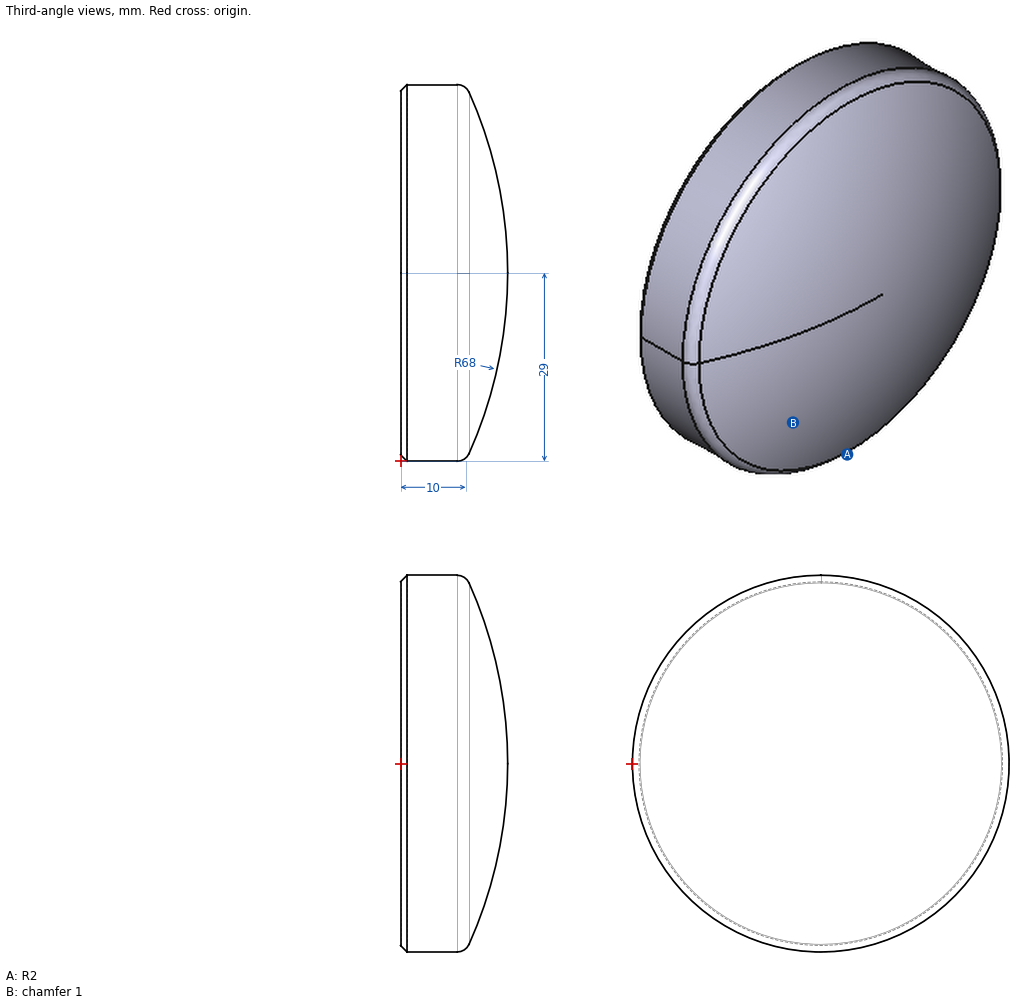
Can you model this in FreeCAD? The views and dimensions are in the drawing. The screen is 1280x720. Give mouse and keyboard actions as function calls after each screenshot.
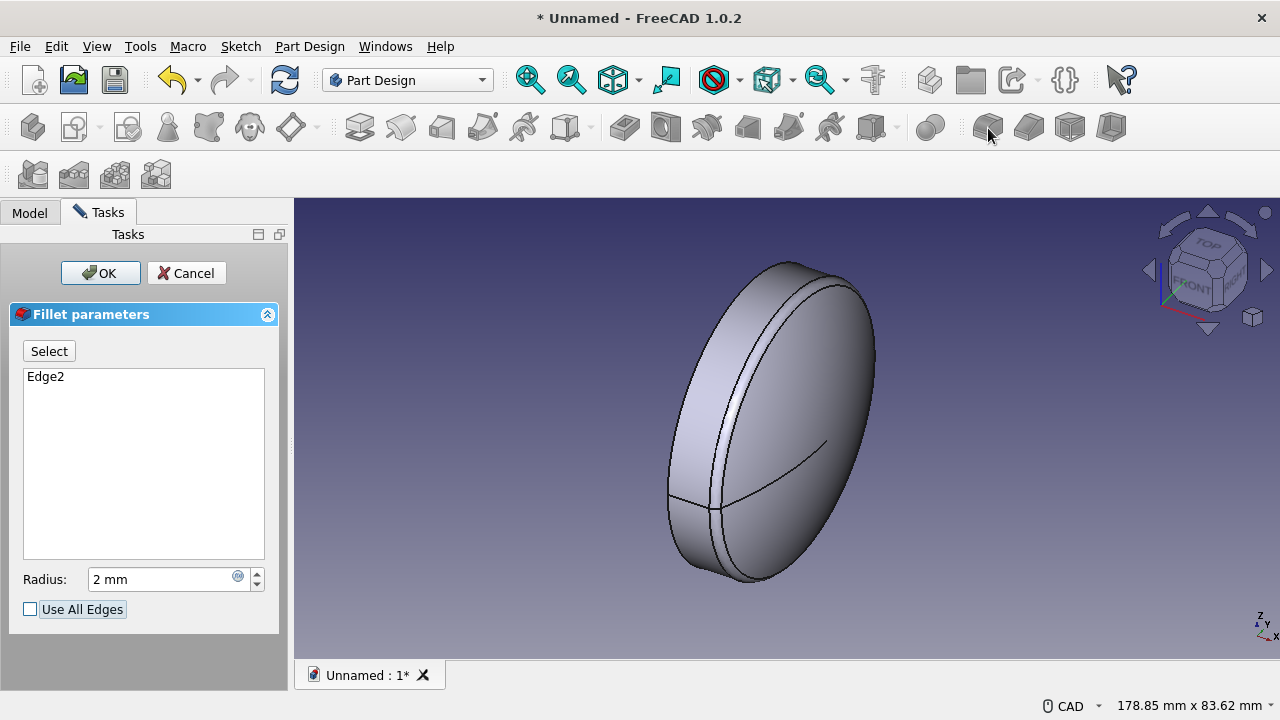
click(101, 273)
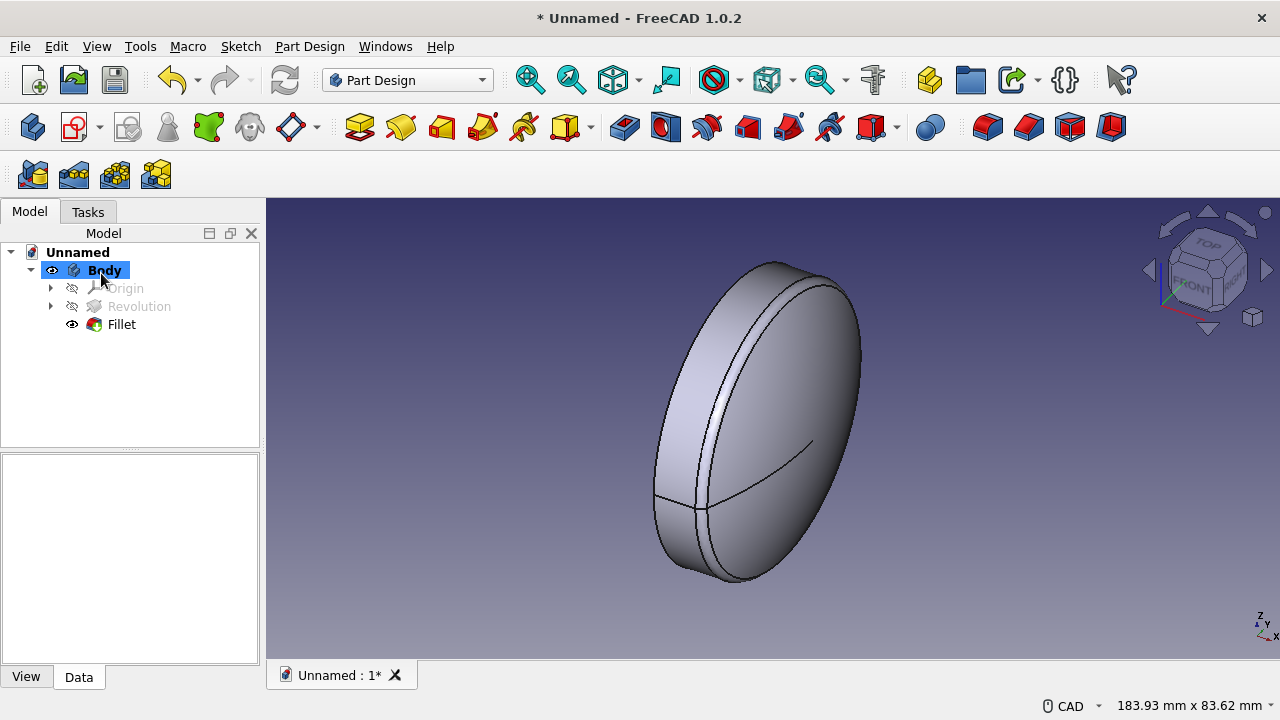
key(0)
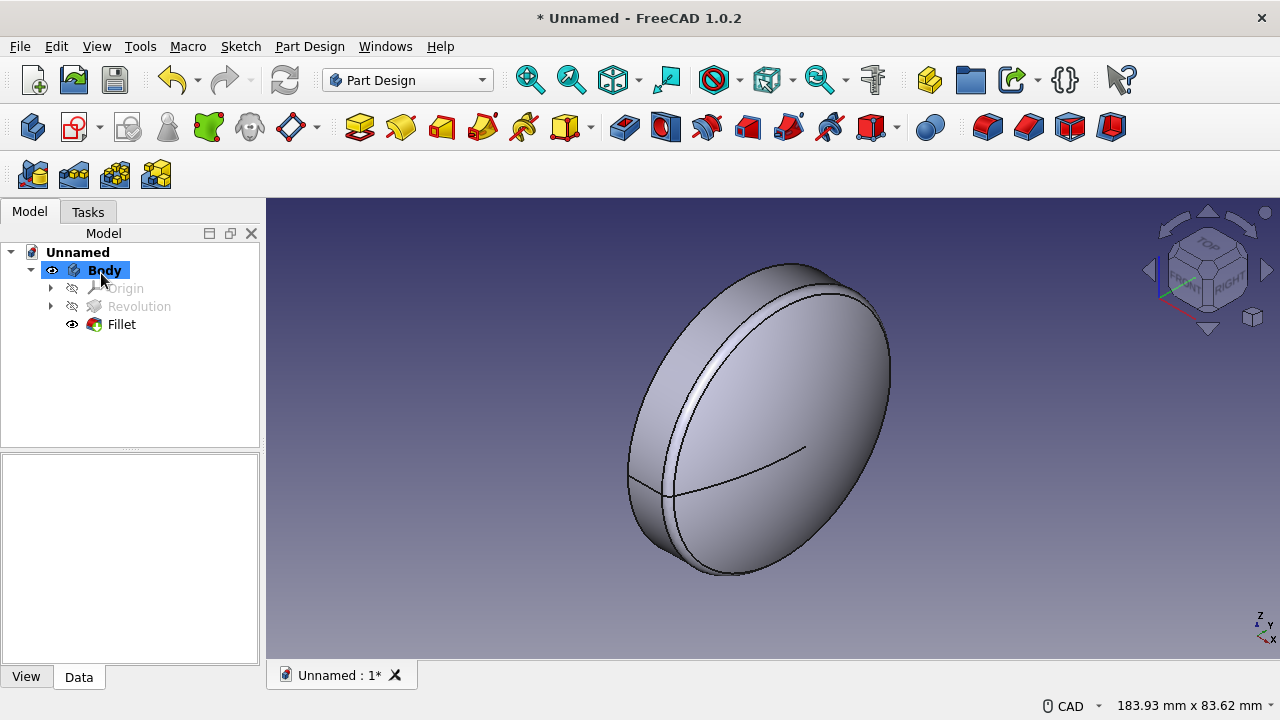
key(2)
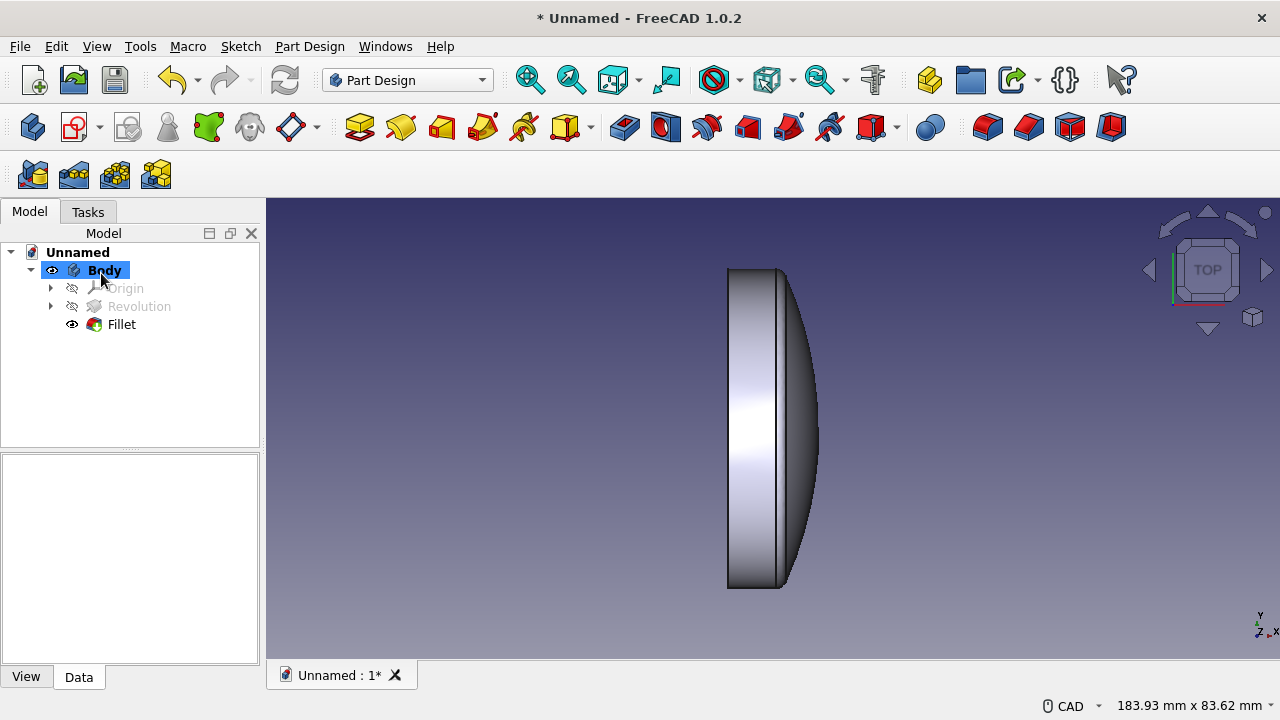
click(728, 378)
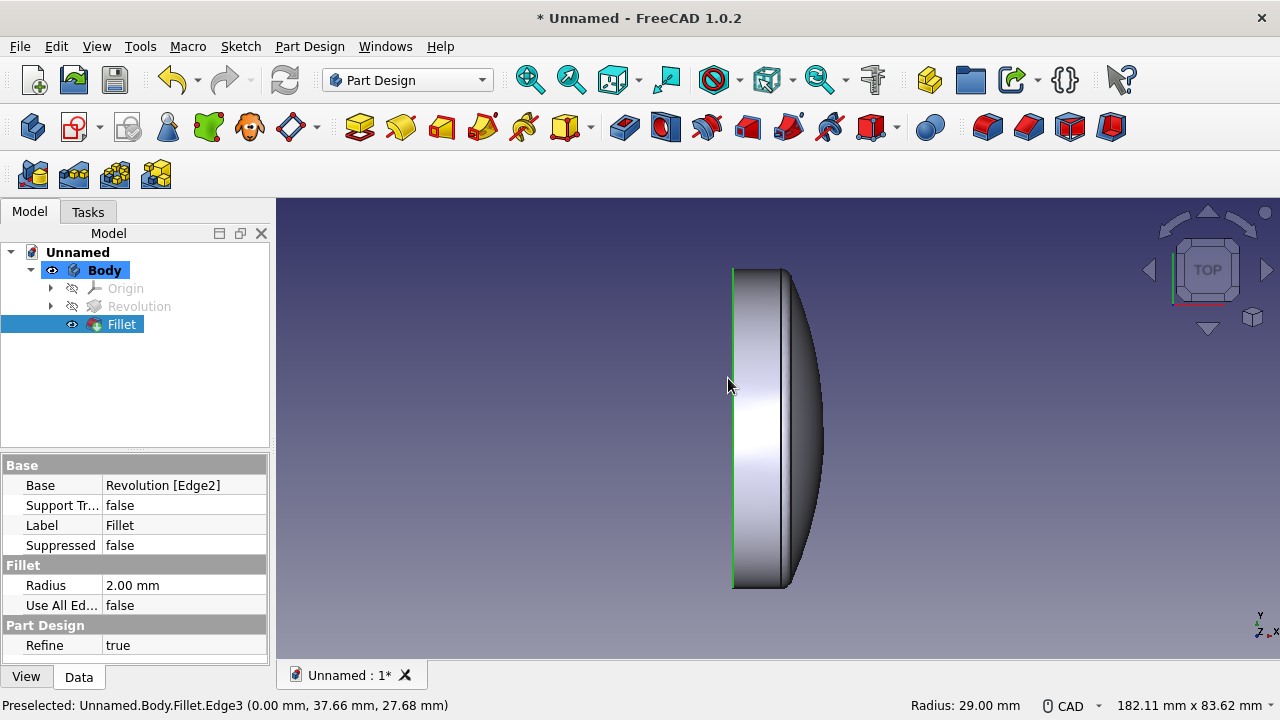
click(1029, 128)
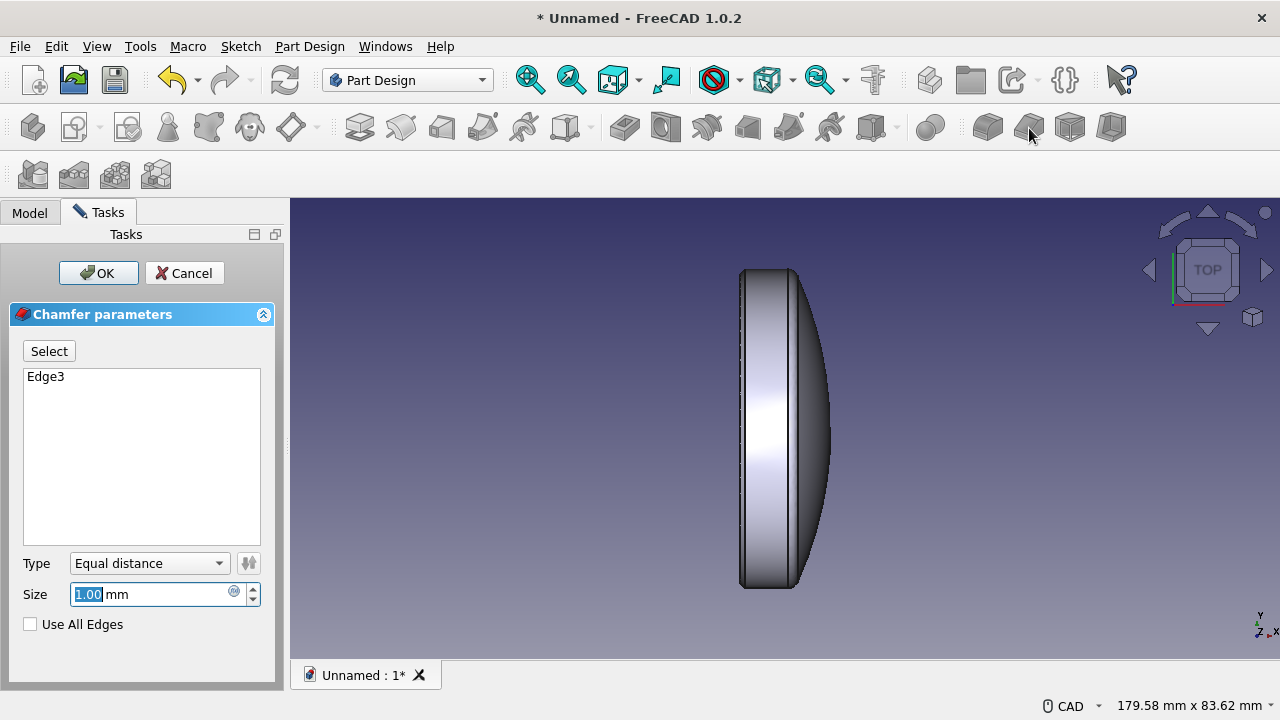
text(1)
key(Tab)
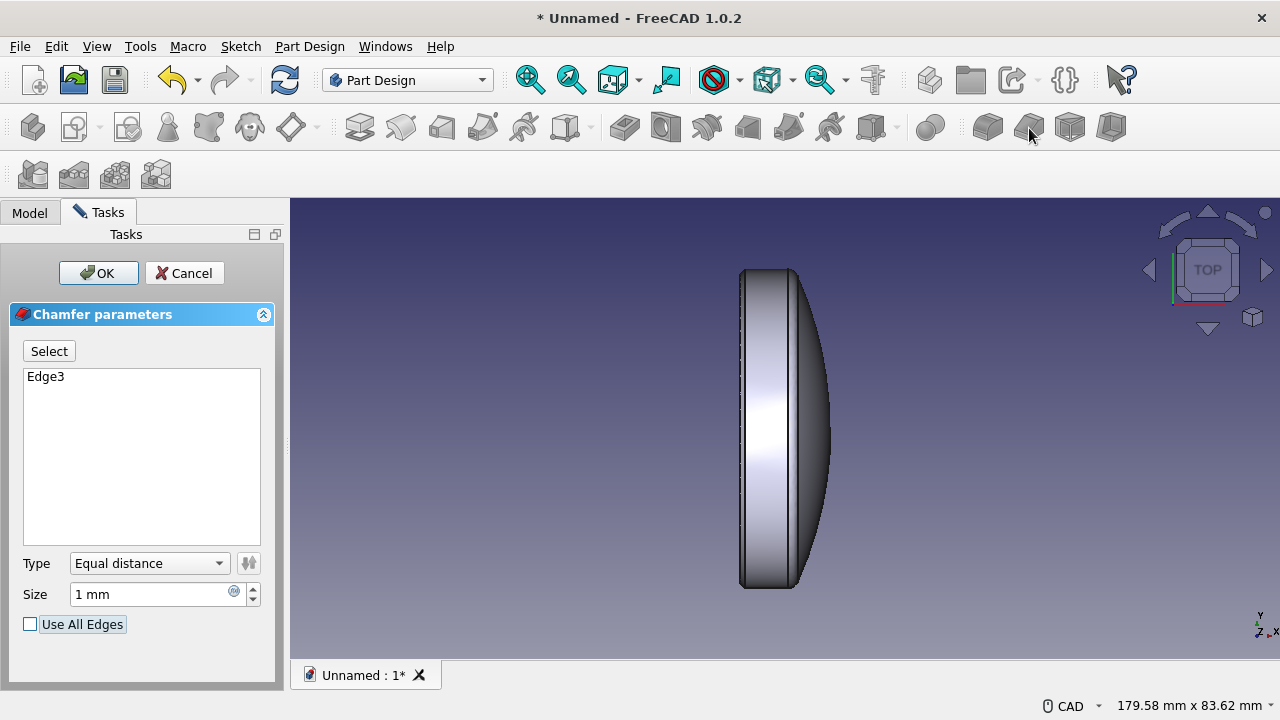
click(99, 273)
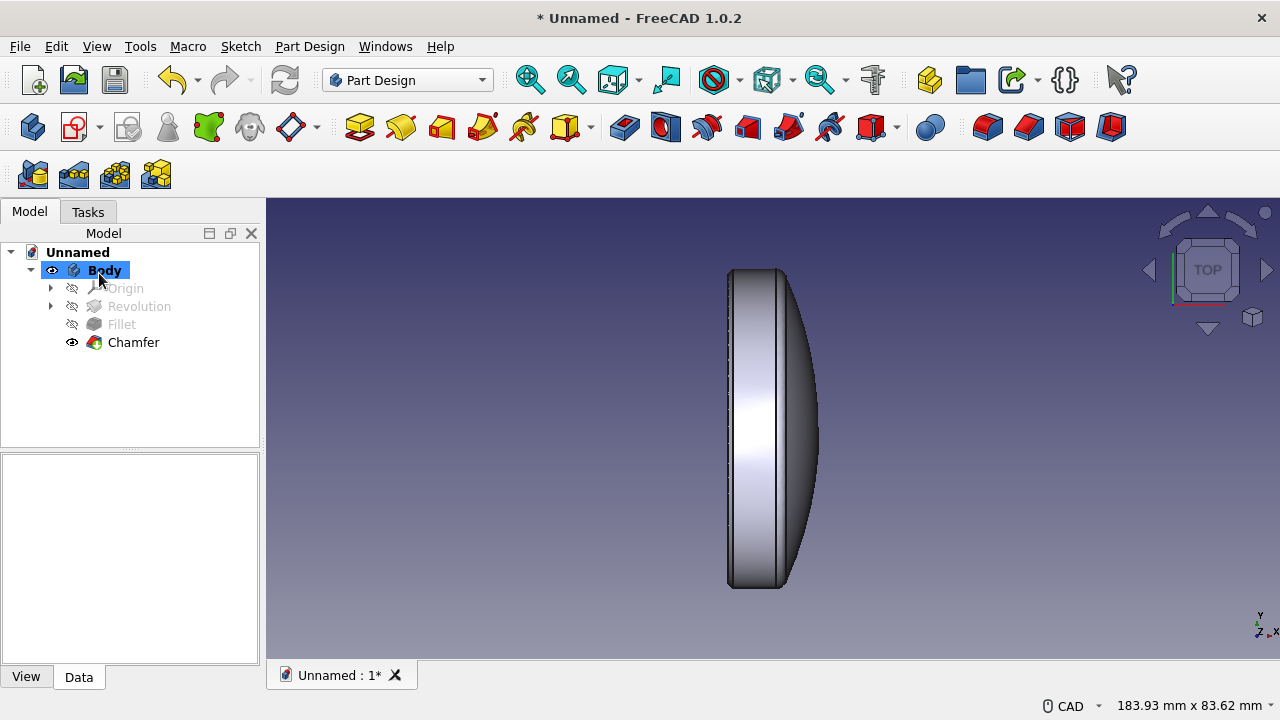
key(0)